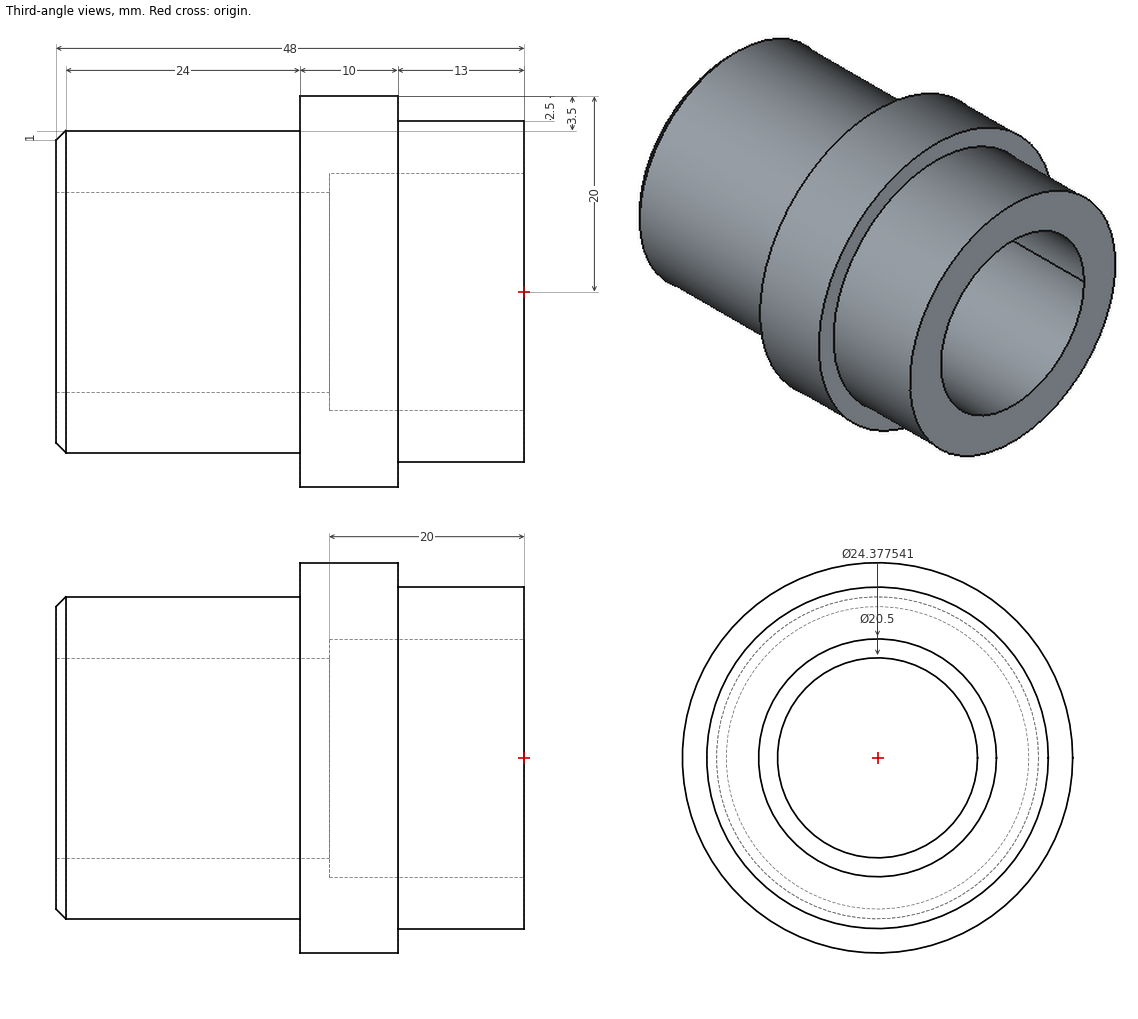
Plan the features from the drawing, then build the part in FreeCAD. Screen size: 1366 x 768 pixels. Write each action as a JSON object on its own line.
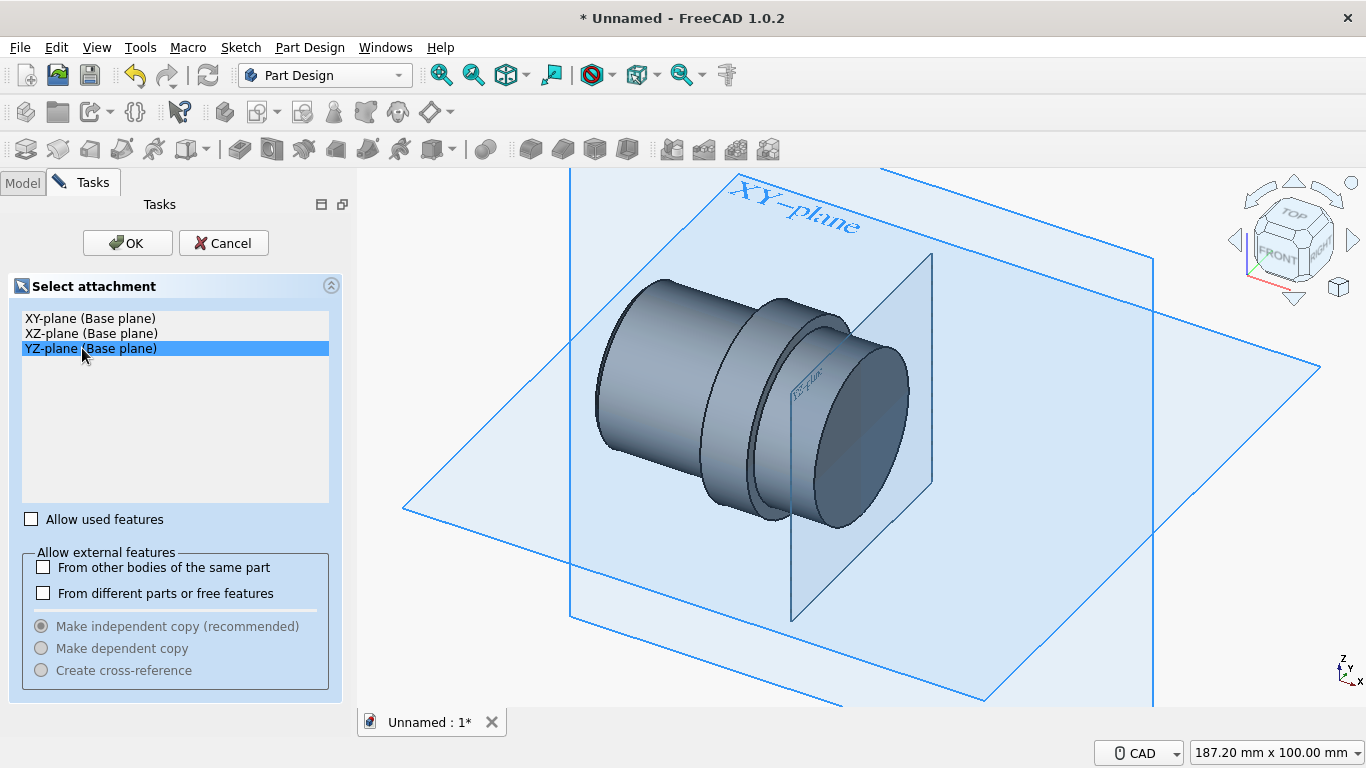
{"action": "left_click", "coordinate": [128, 243]}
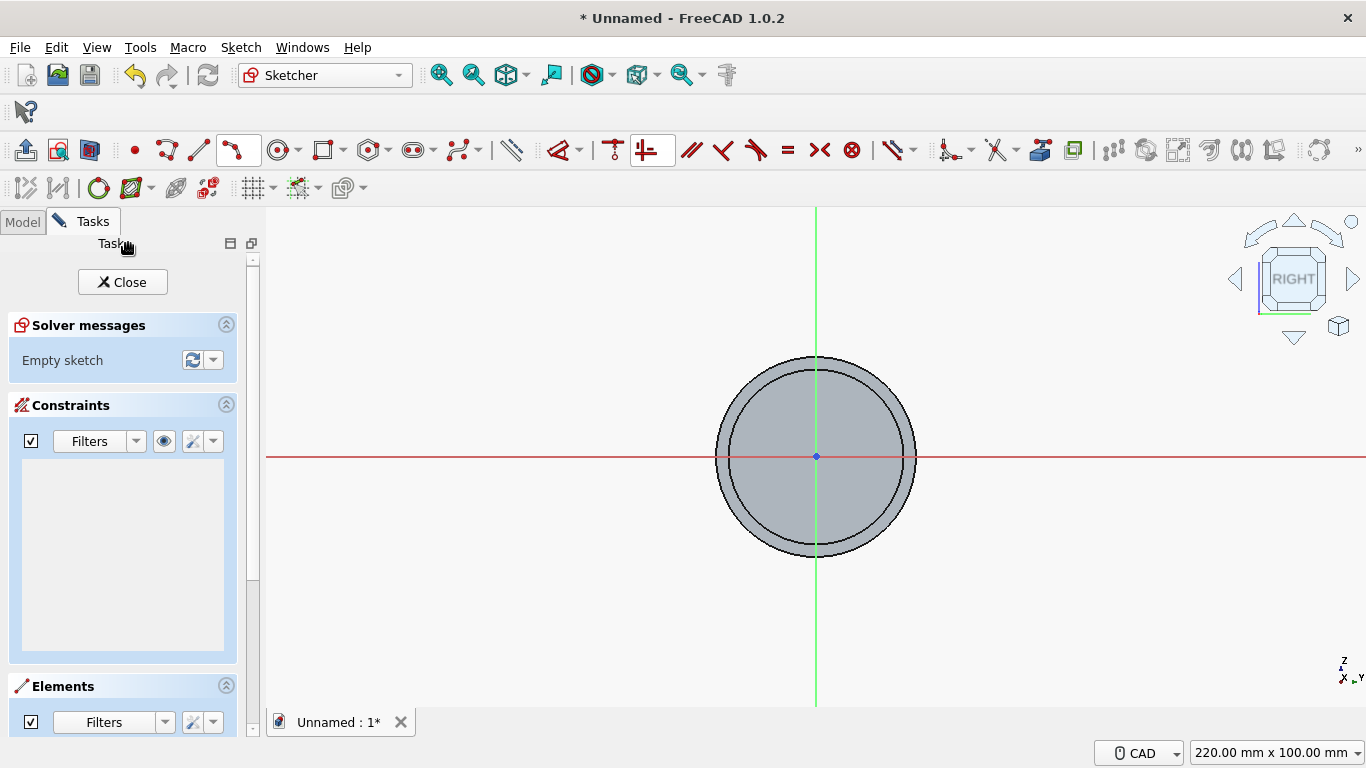
{"action": "scroll", "coordinate": [846, 457], "scroll_direction": "up", "scroll_amount": 6}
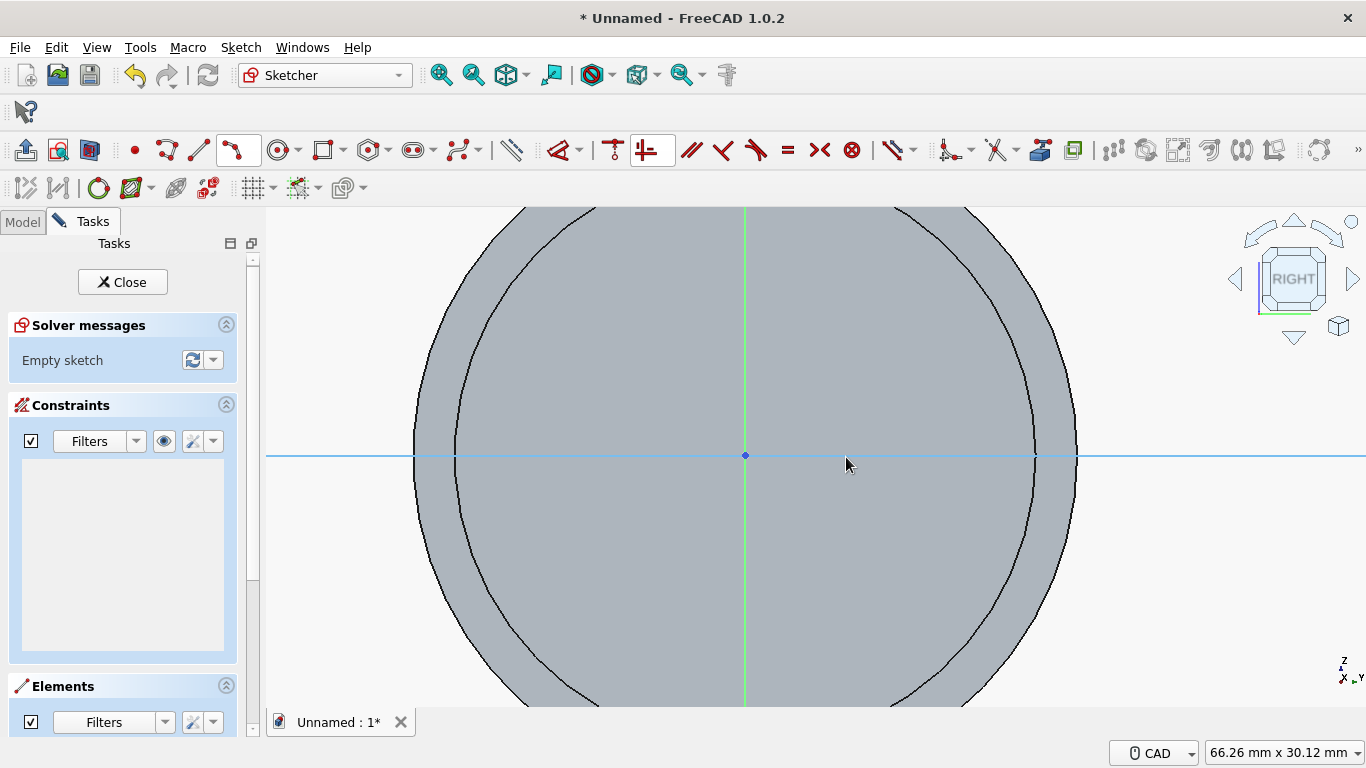
{"action": "left_click", "coordinate": [278, 150]}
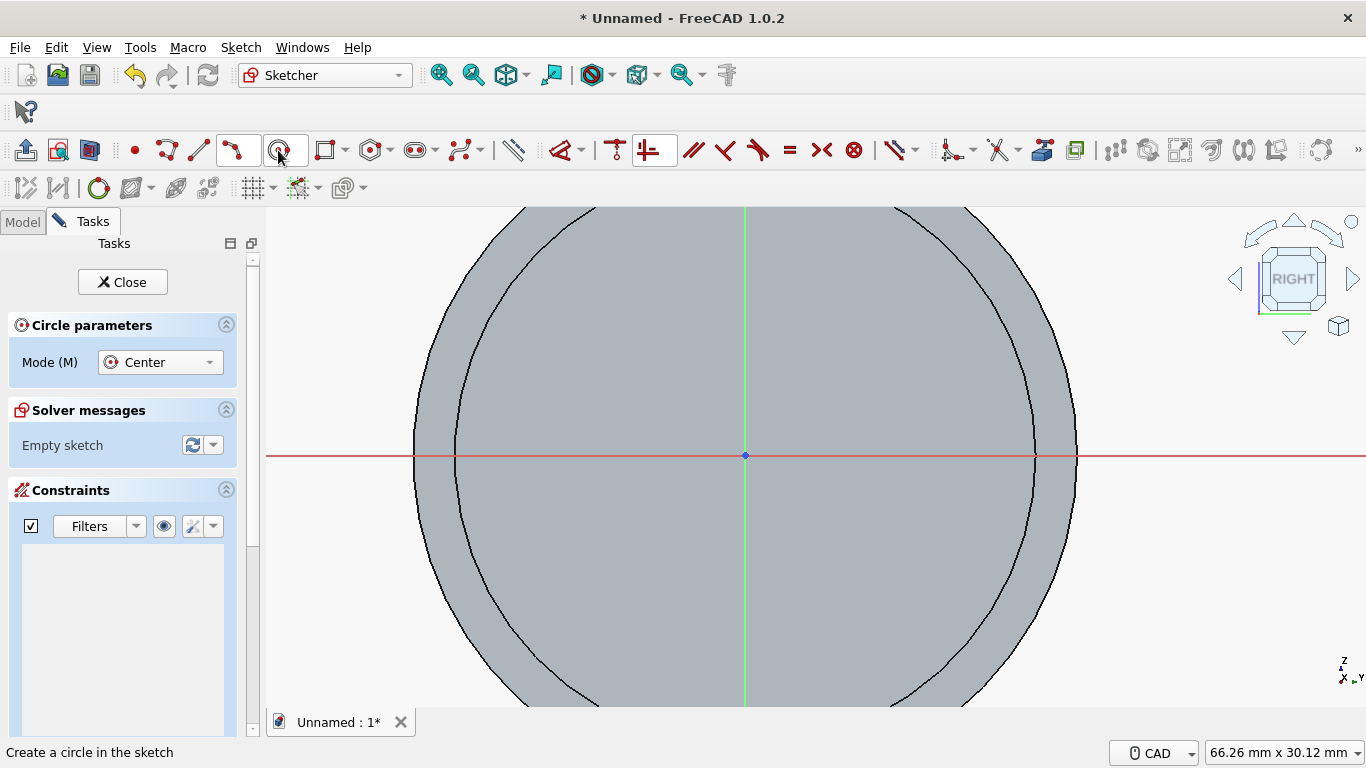
{"action": "left_click", "coordinate": [745, 456]}
{"action": "mouse_move", "coordinate": [865, 336]}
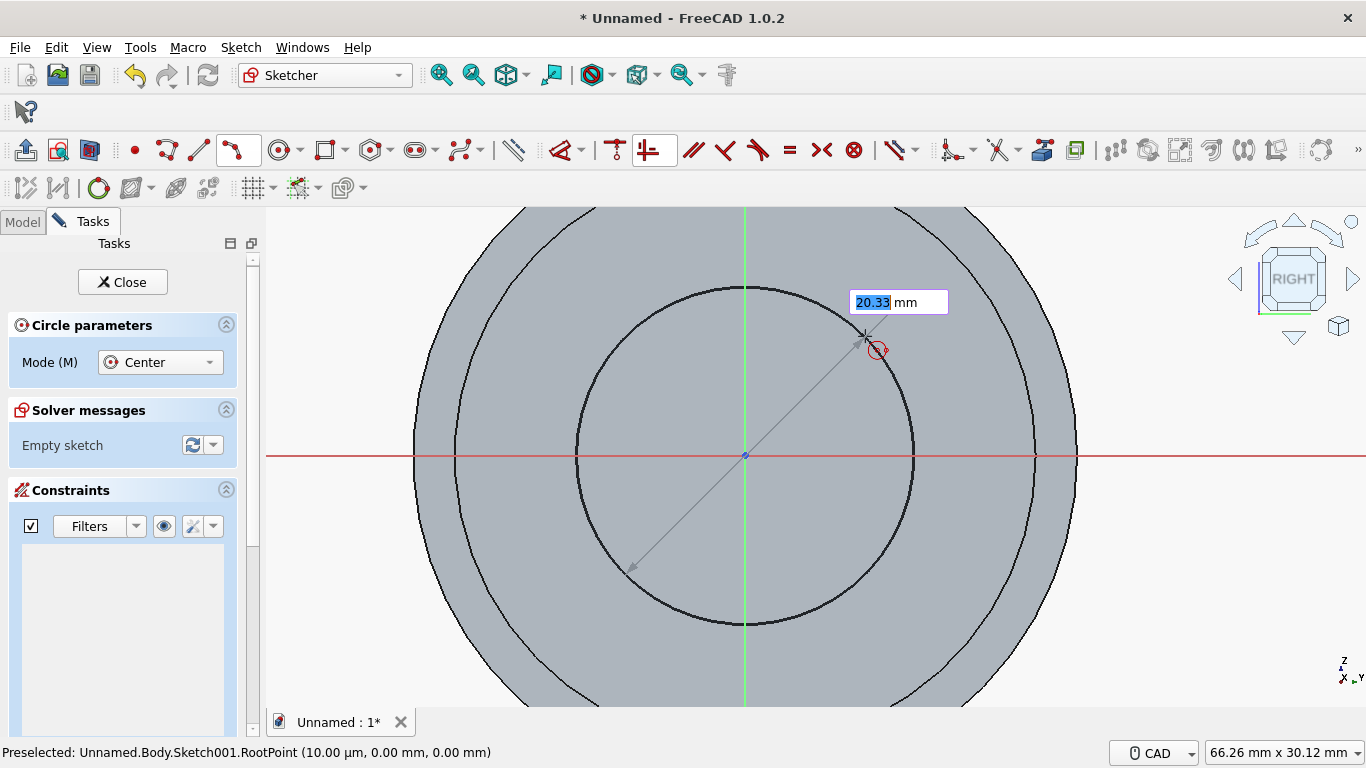
{"action": "type", "text": "20.5"}
{"action": "key", "text": "Return"}
{"action": "key", "text": "Escape"}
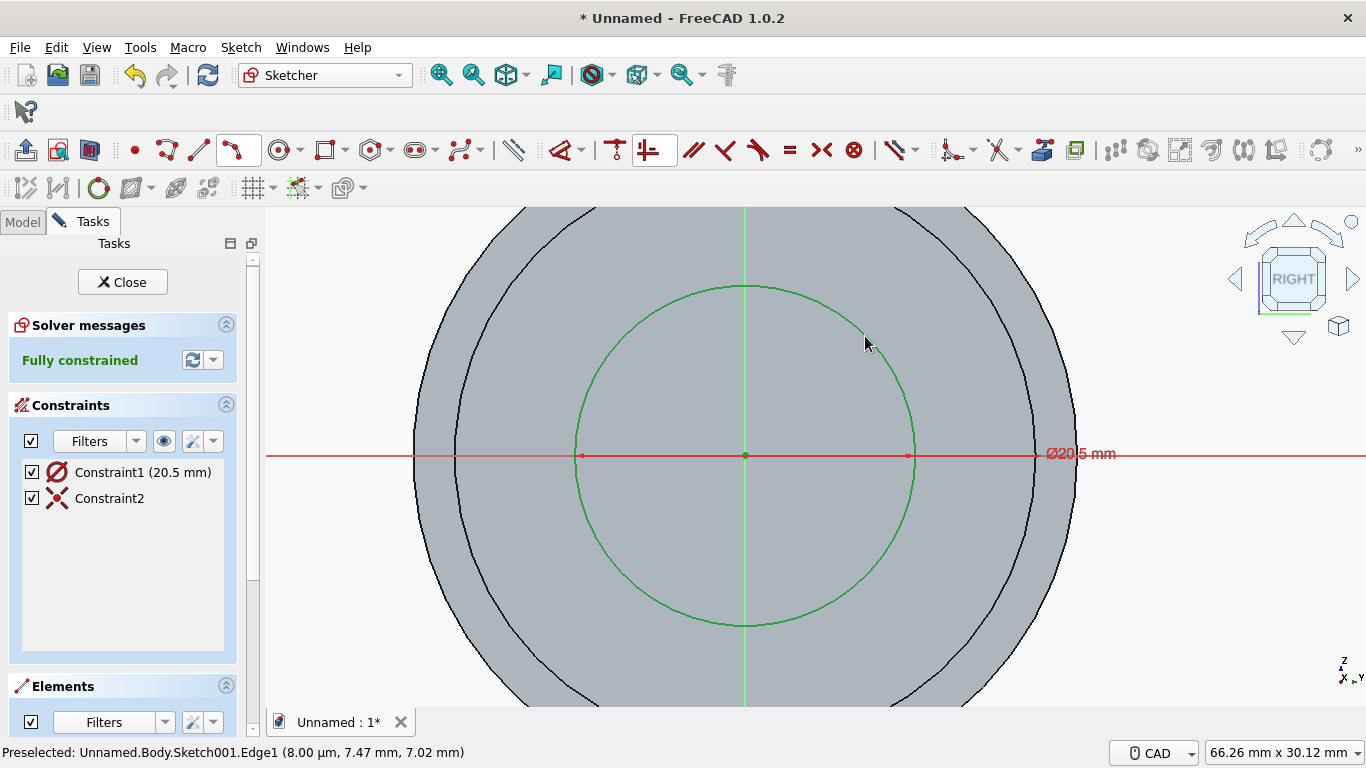
{"action": "left_click", "coordinate": [123, 282]}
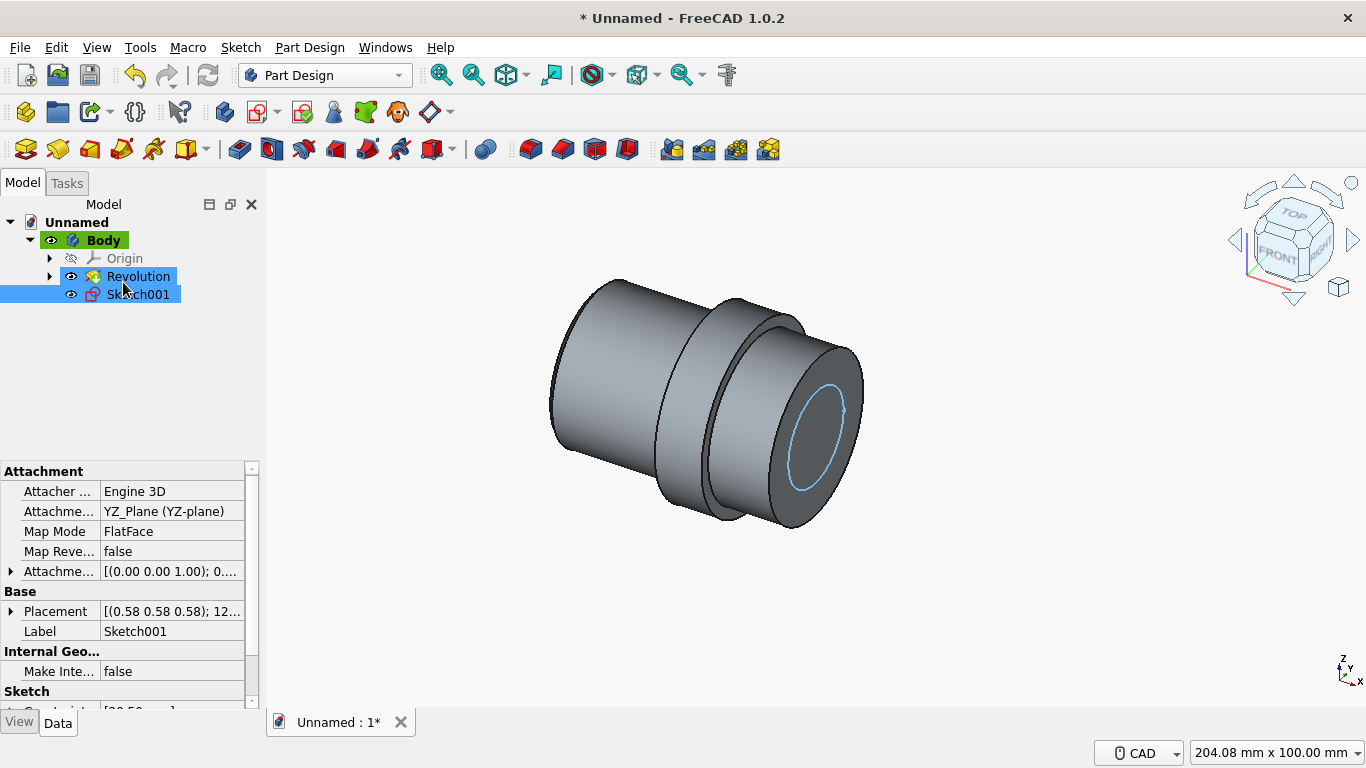
{"action": "left_click", "coordinate": [240, 150]}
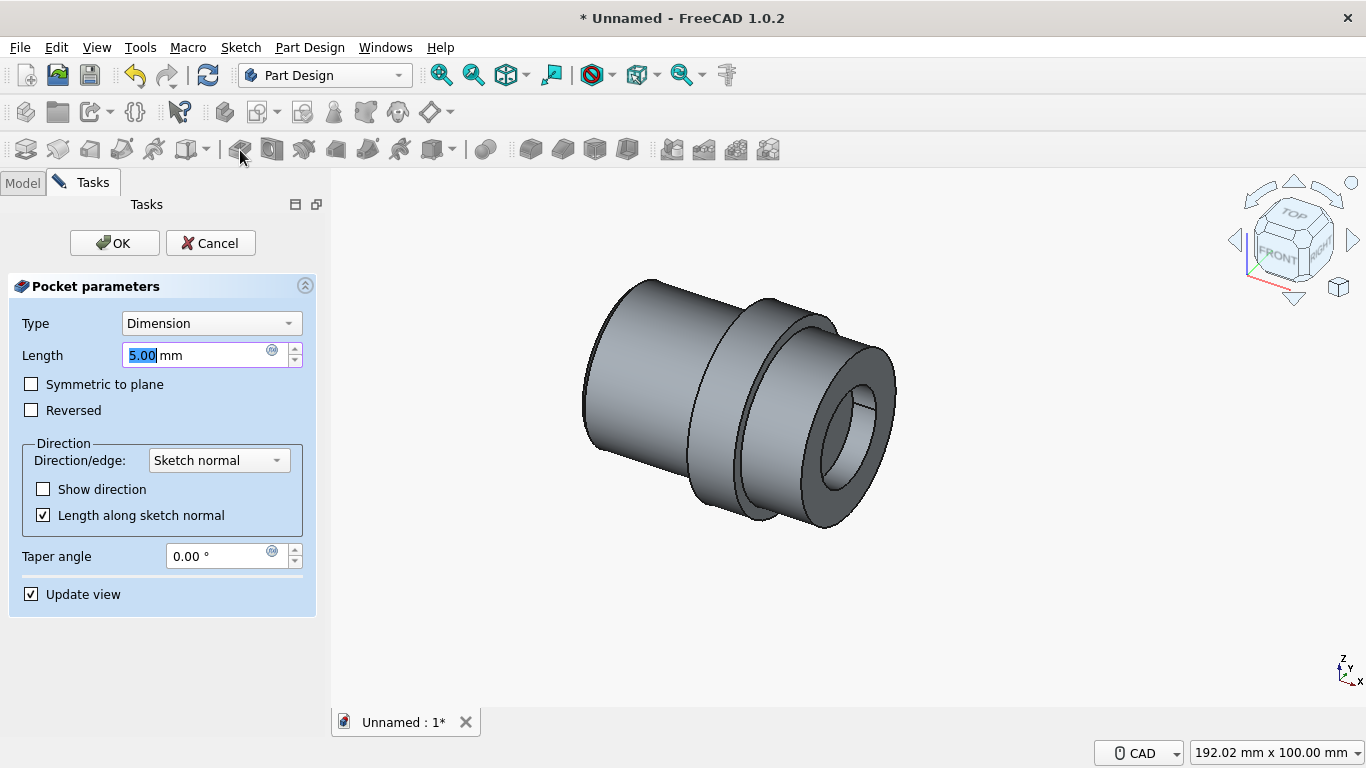
{"action": "left_click", "coordinate": [212, 324]}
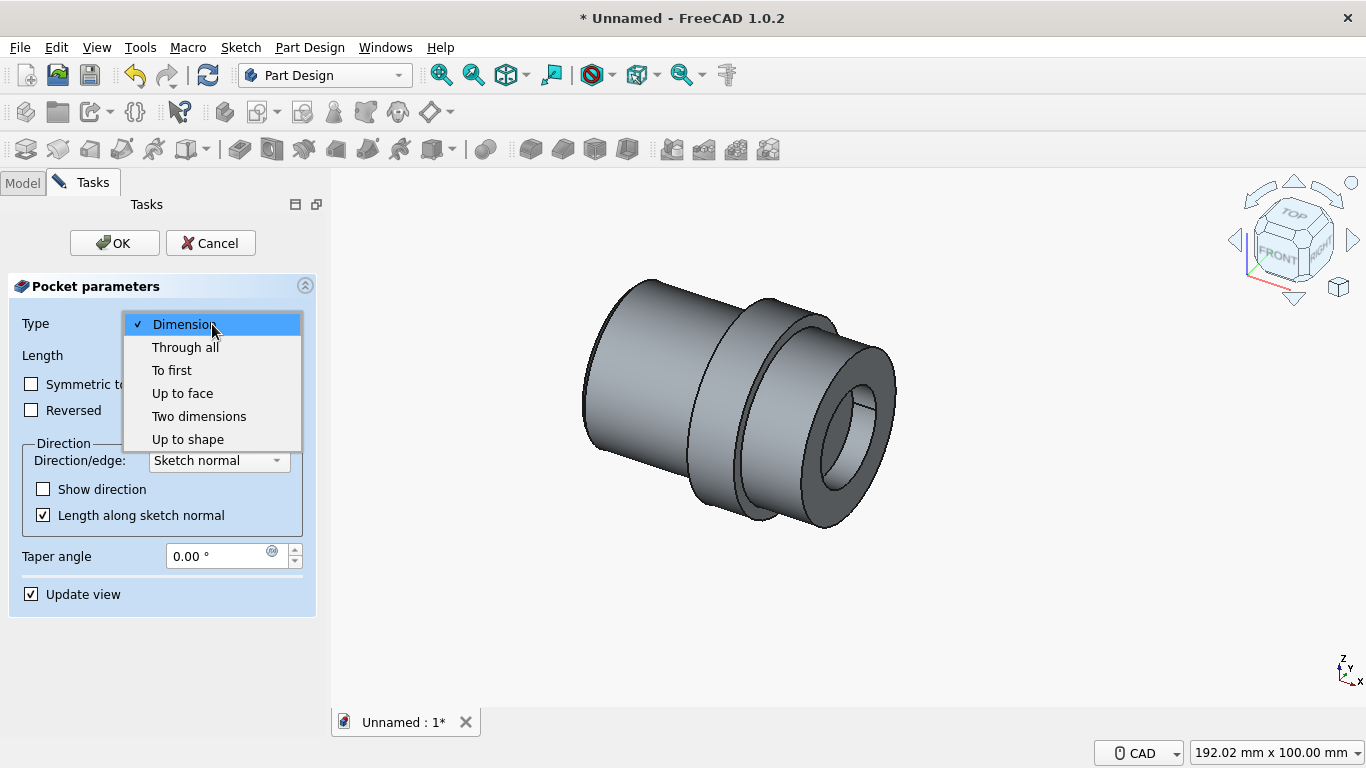
{"action": "left_click", "coordinate": [212, 348]}